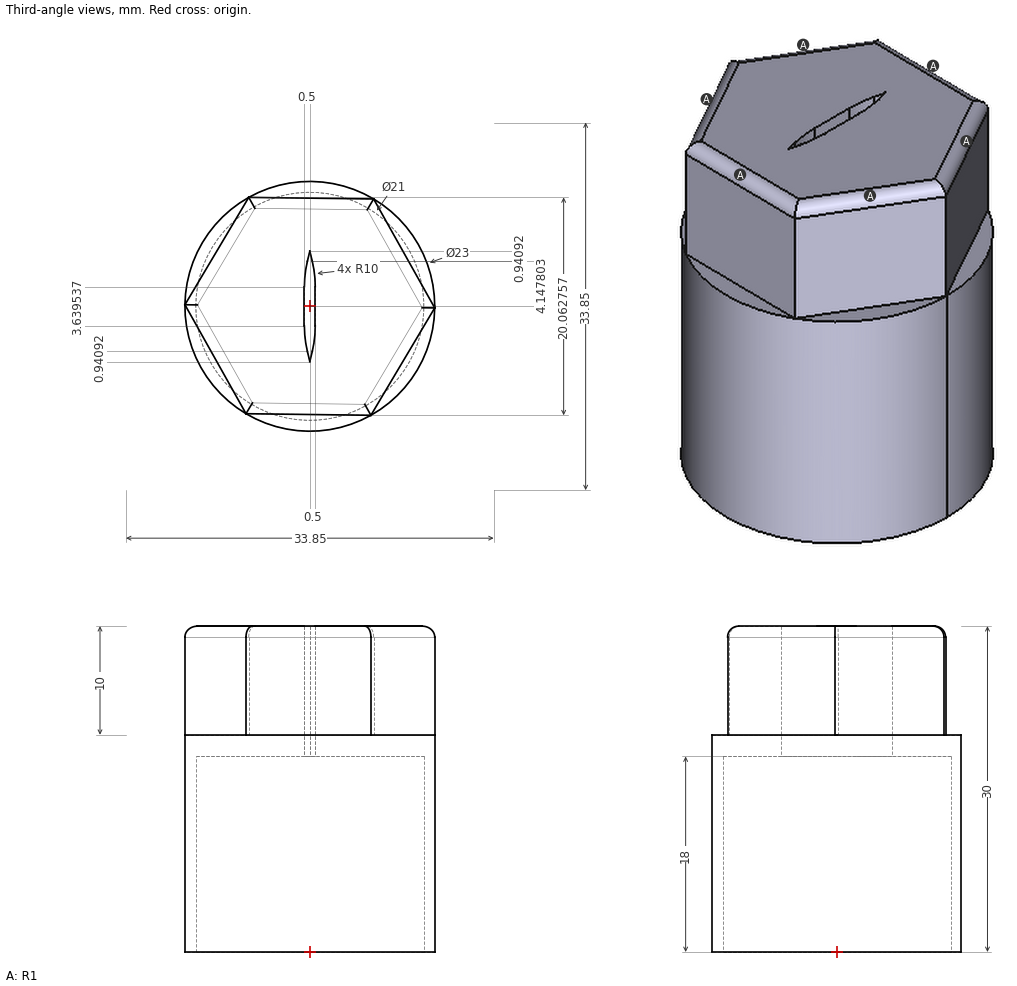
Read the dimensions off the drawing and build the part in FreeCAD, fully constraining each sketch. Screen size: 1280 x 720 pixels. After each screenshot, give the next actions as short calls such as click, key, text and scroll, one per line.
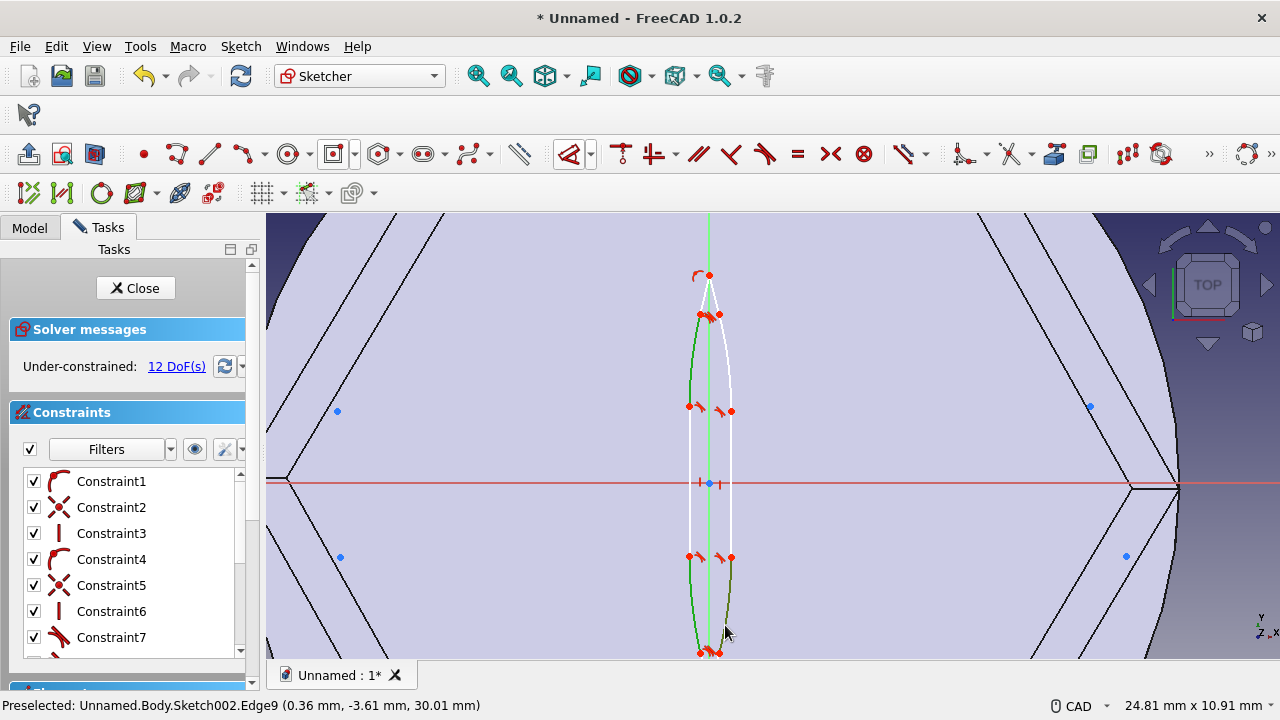
click(730, 382)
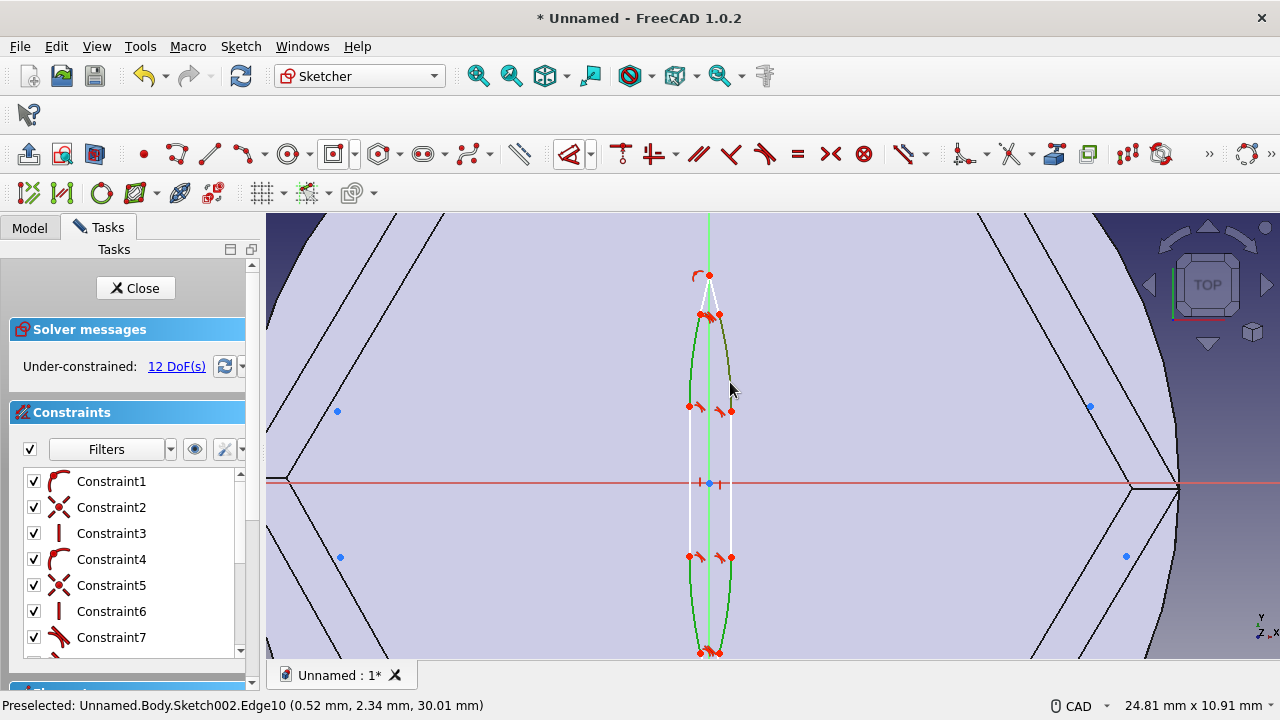
click(798, 154)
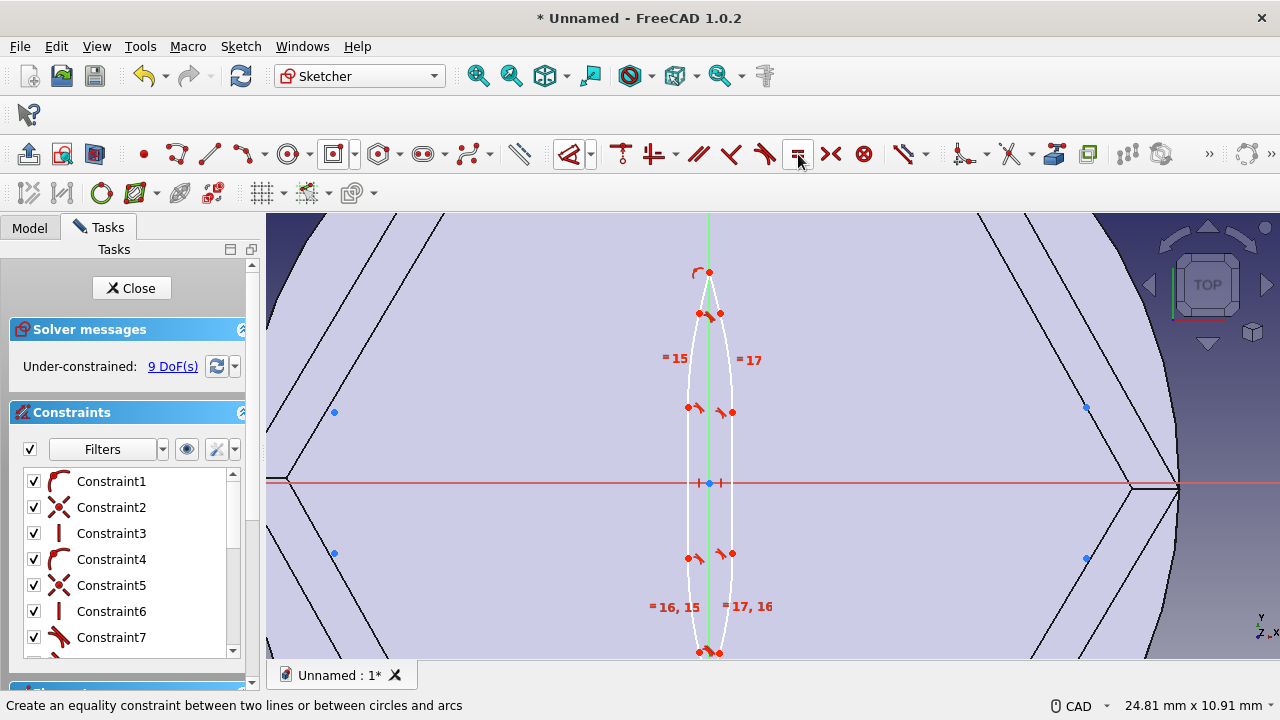
click(694, 342)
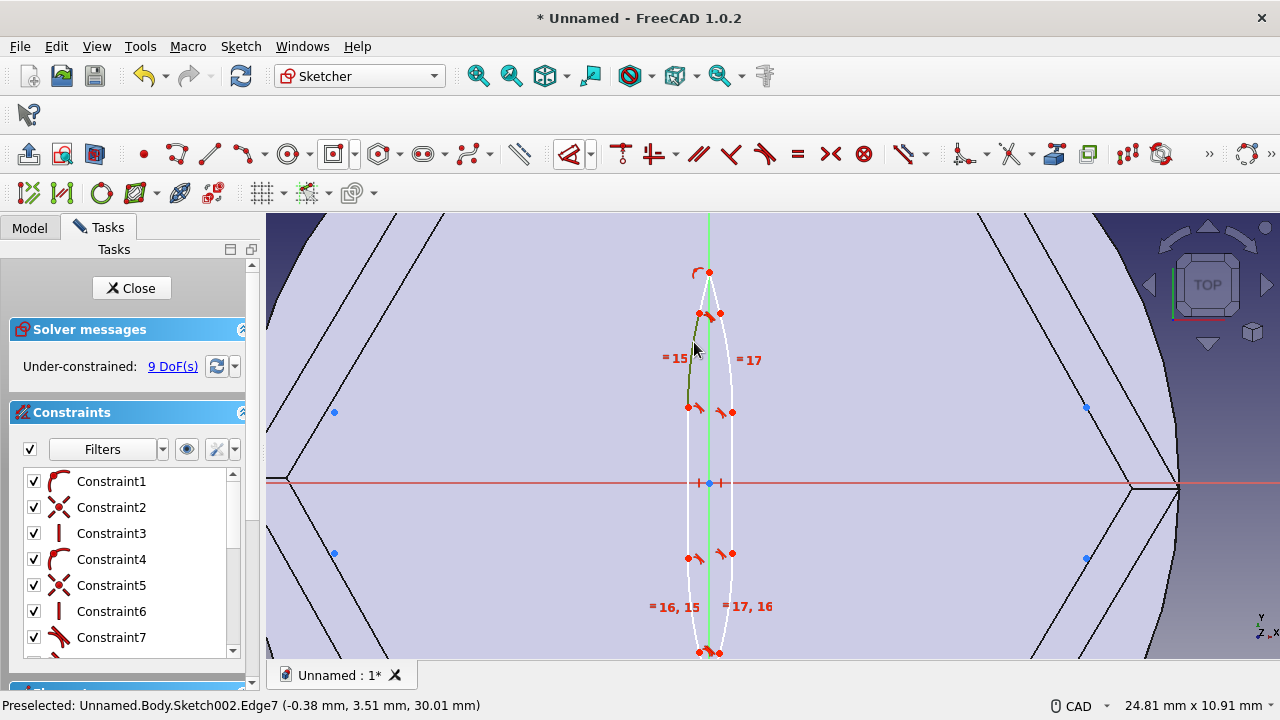
click(590, 154)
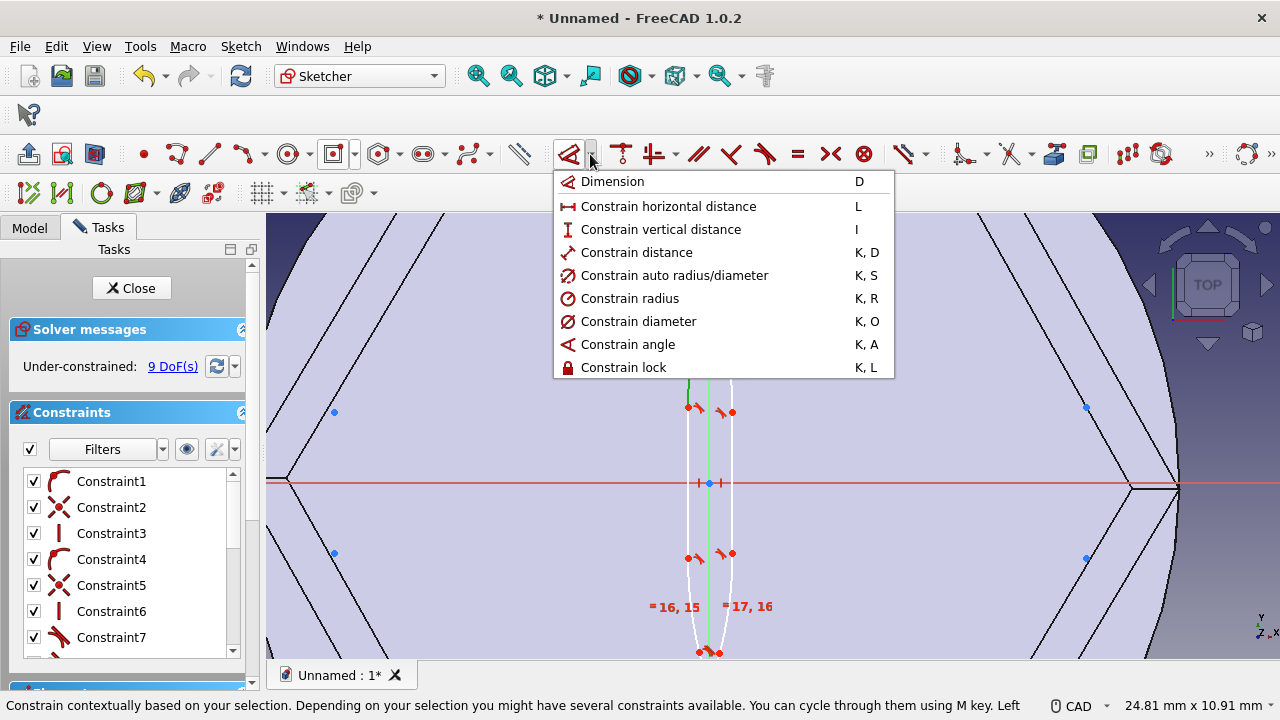
click(724, 298)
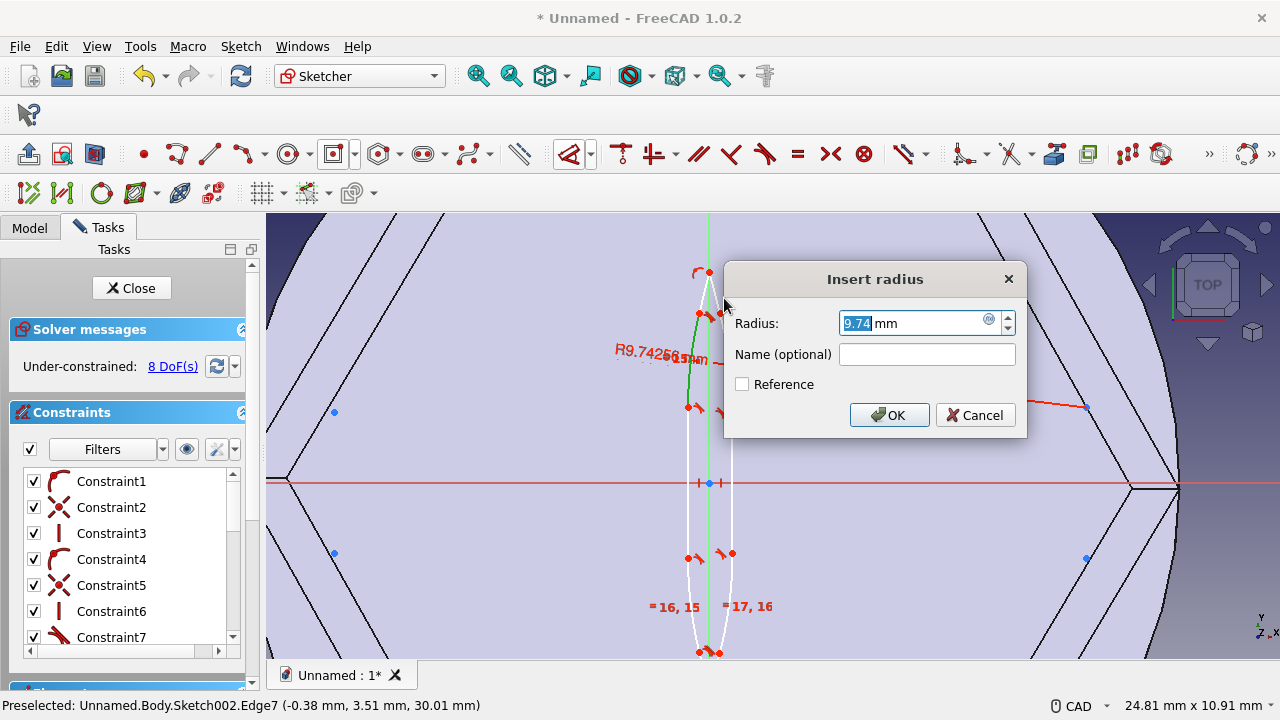
text(10)
key(Return)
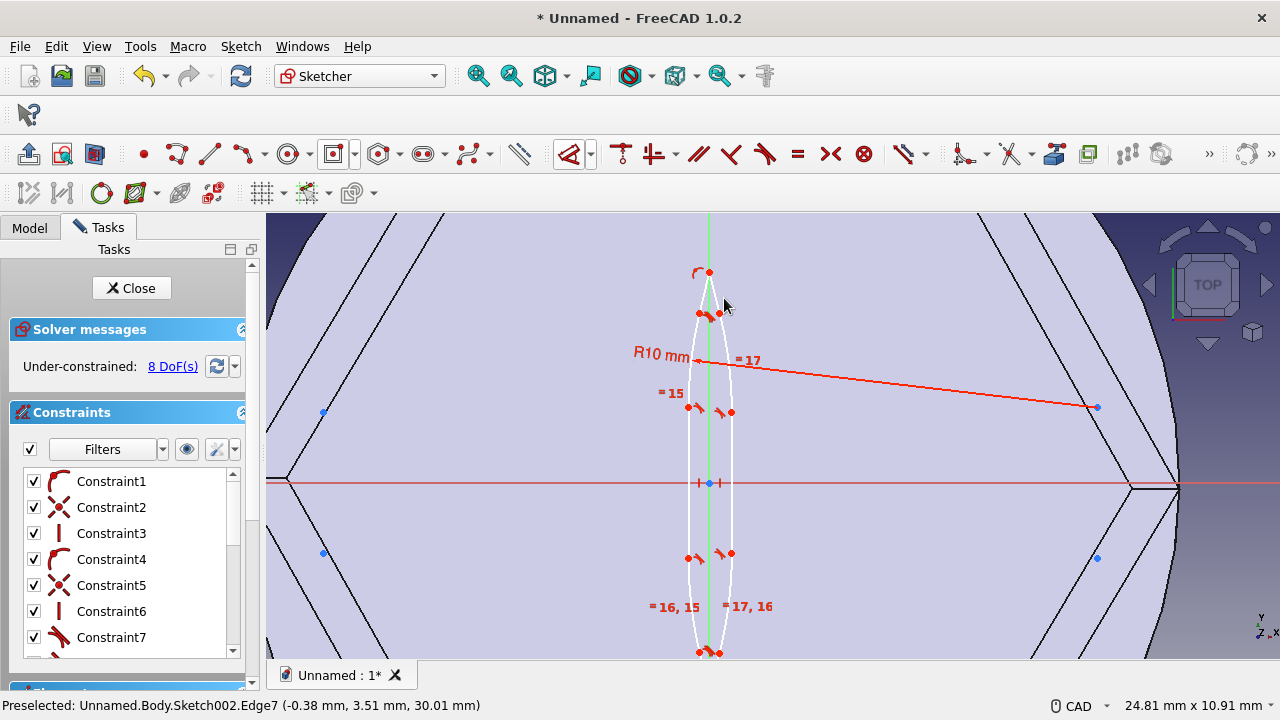
scroll(689, 408, up, 4)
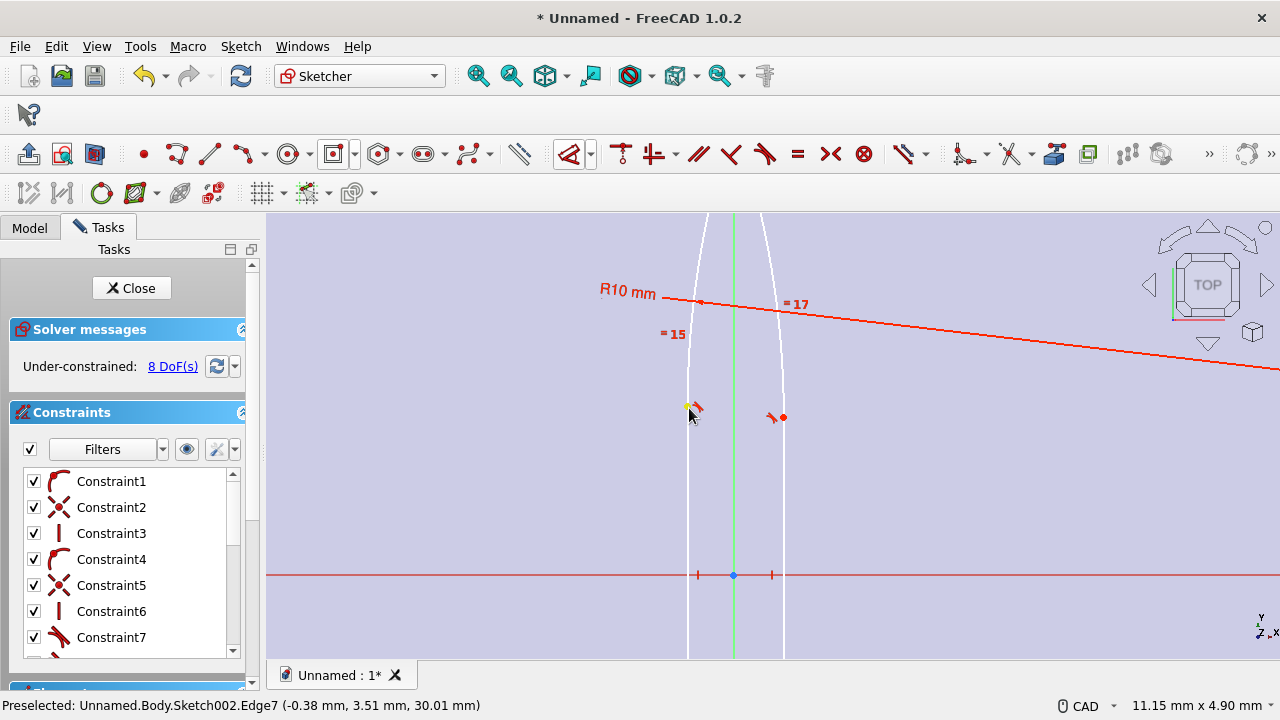
click(688, 407)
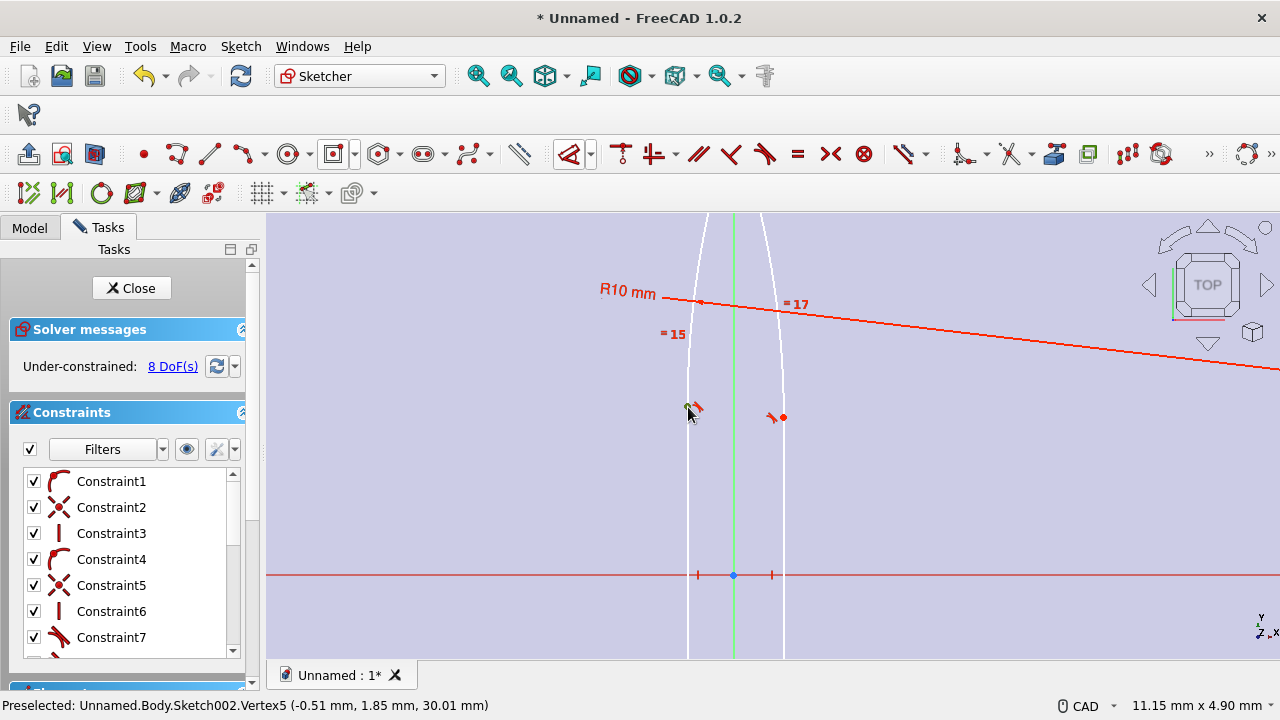
key(l)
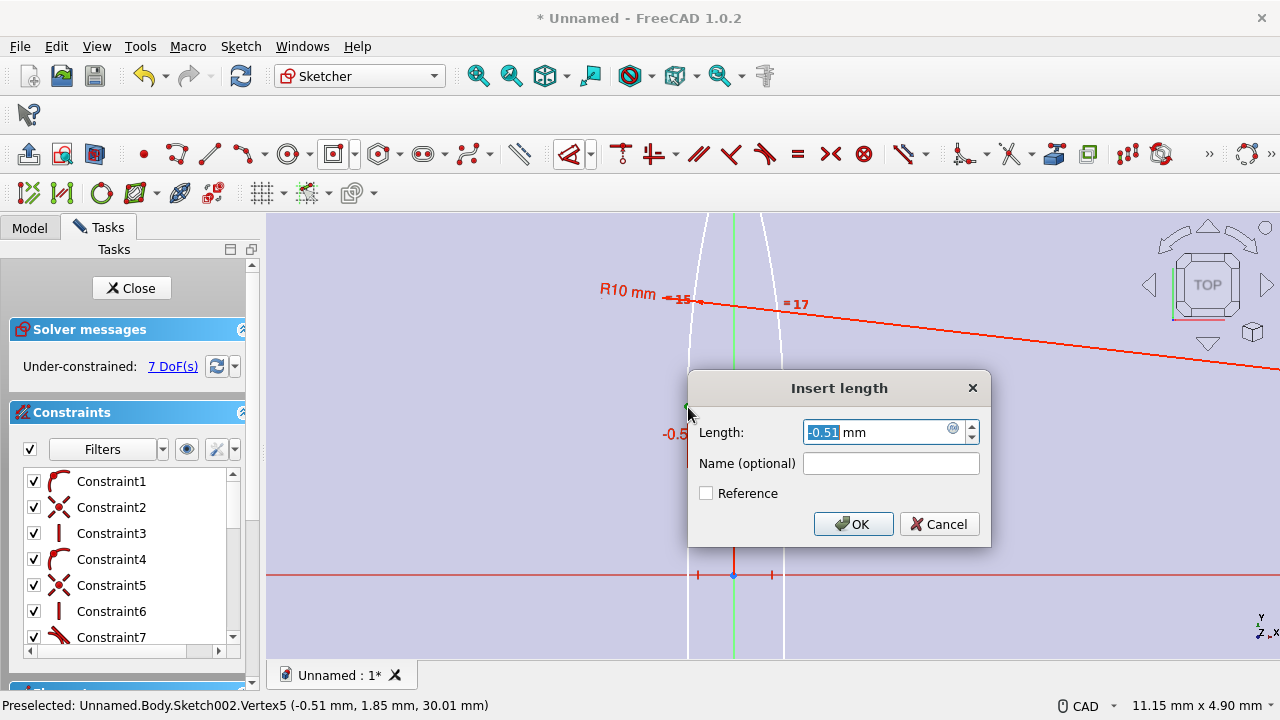
text(-0.5)
key(Return)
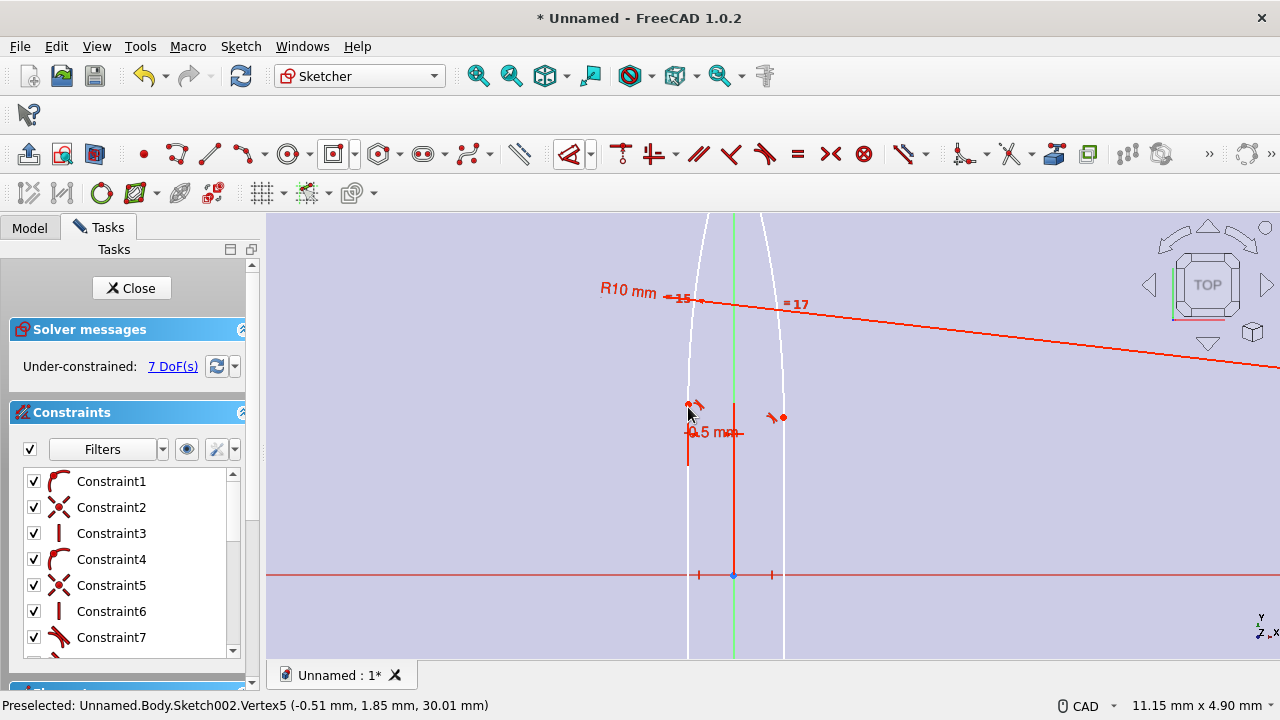
scroll(692, 376, down, 6)